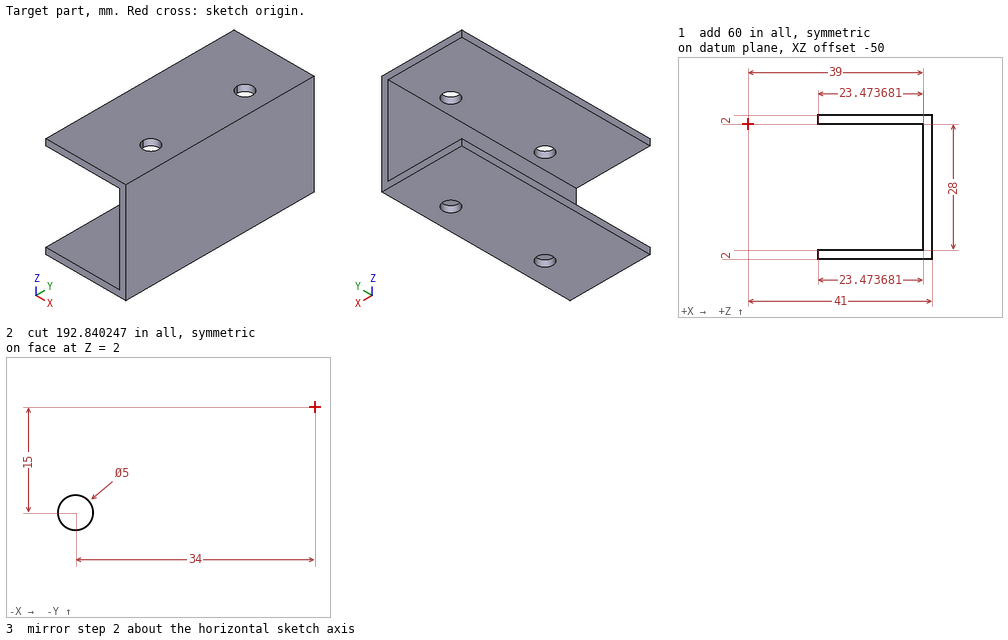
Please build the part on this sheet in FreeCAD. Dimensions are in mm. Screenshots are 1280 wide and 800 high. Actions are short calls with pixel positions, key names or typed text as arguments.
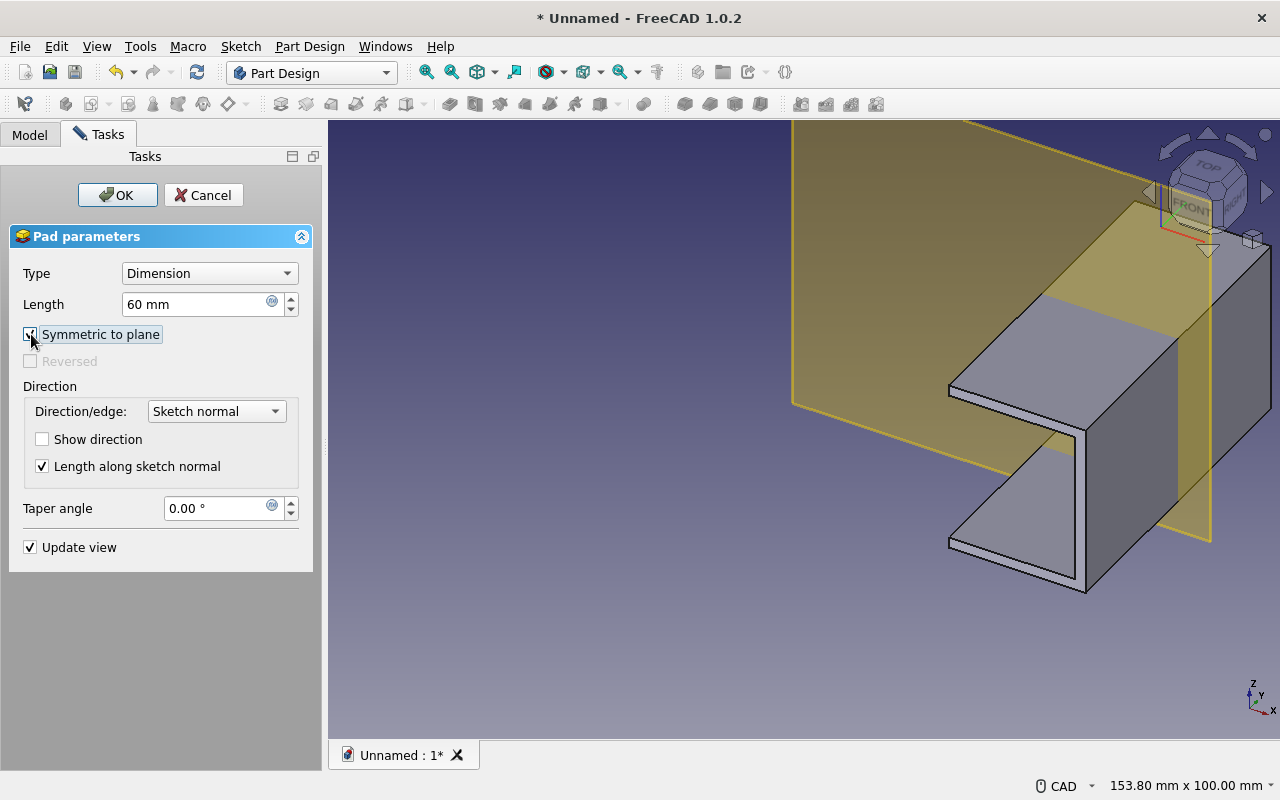
click(118, 195)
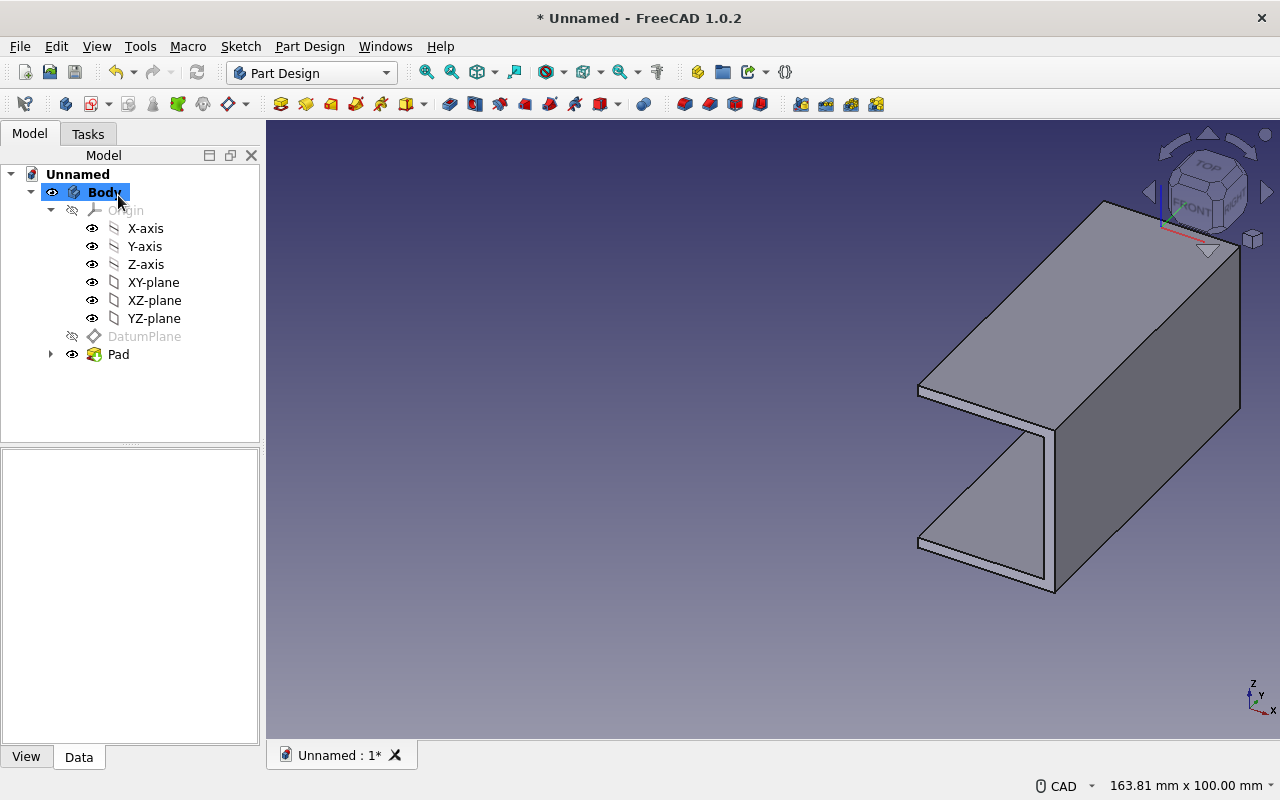
click(1106, 288)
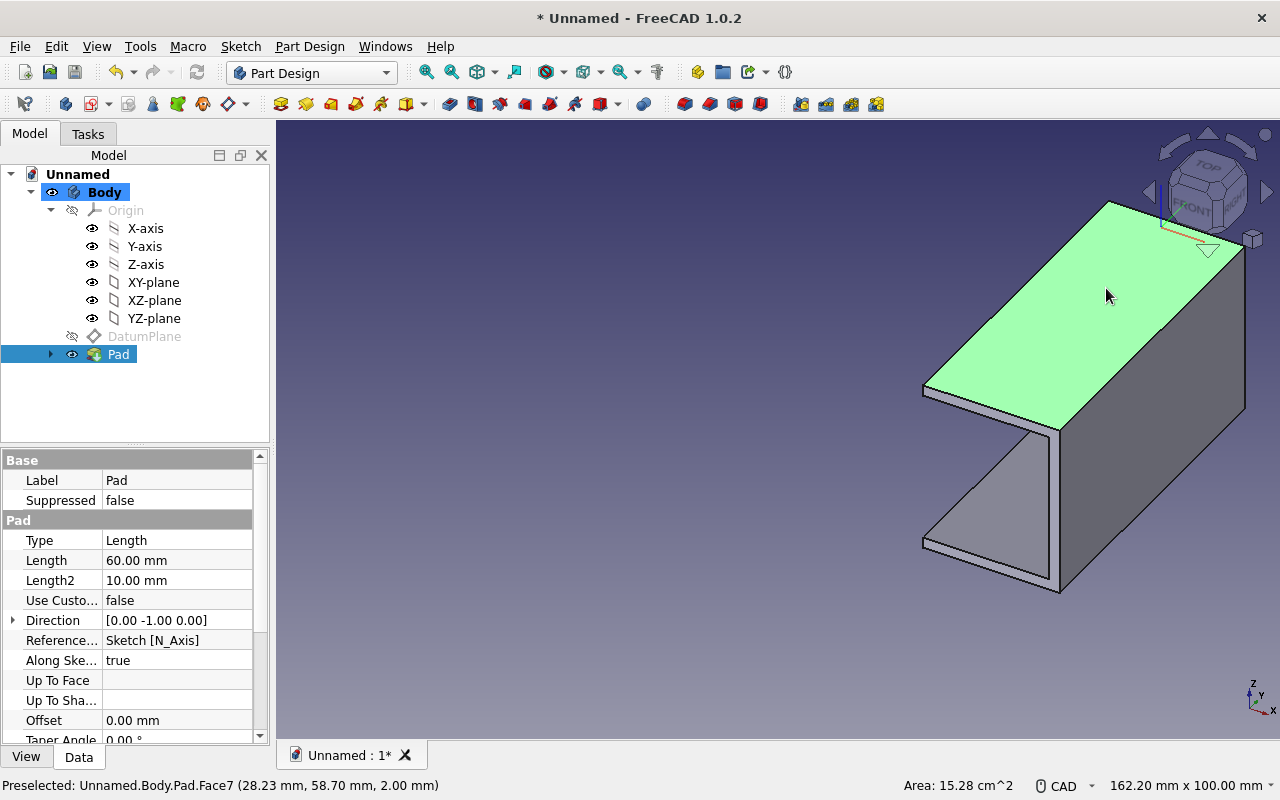
click(90, 104)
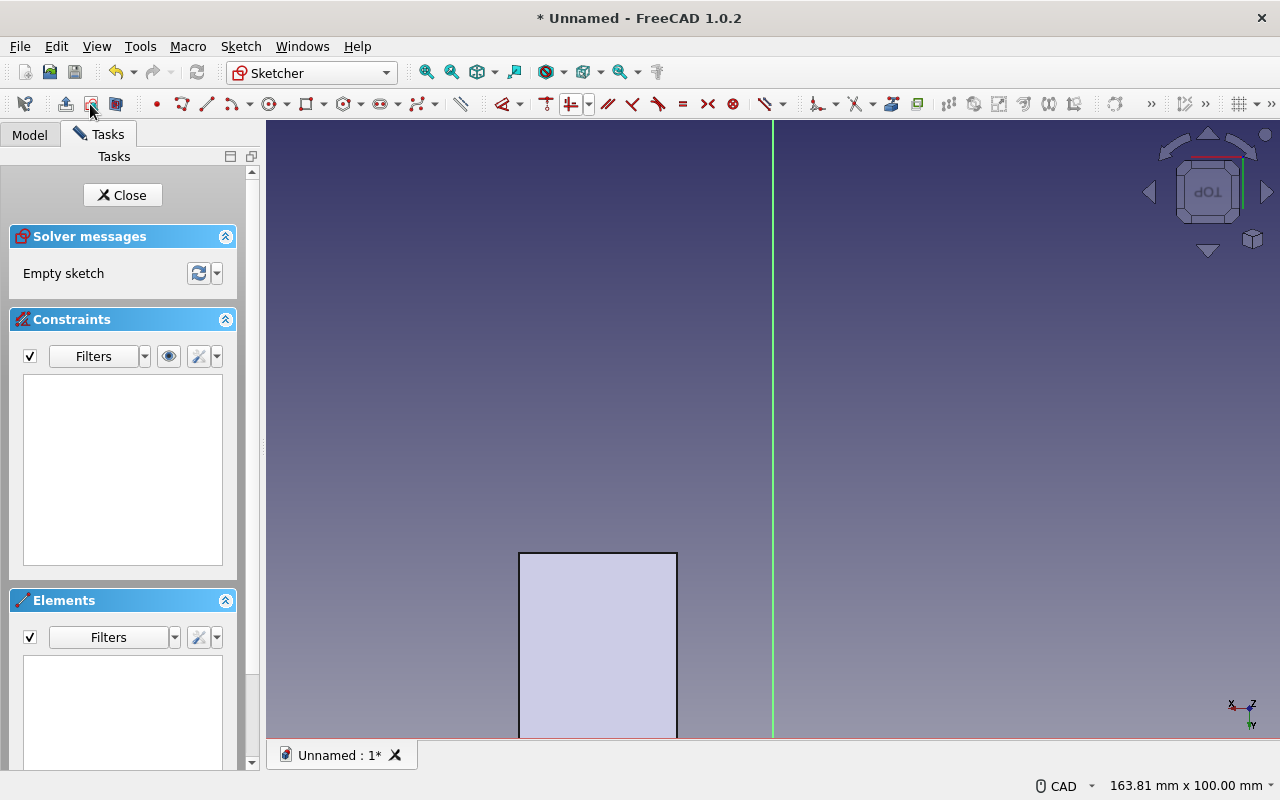
scroll(704, 430, down, 5)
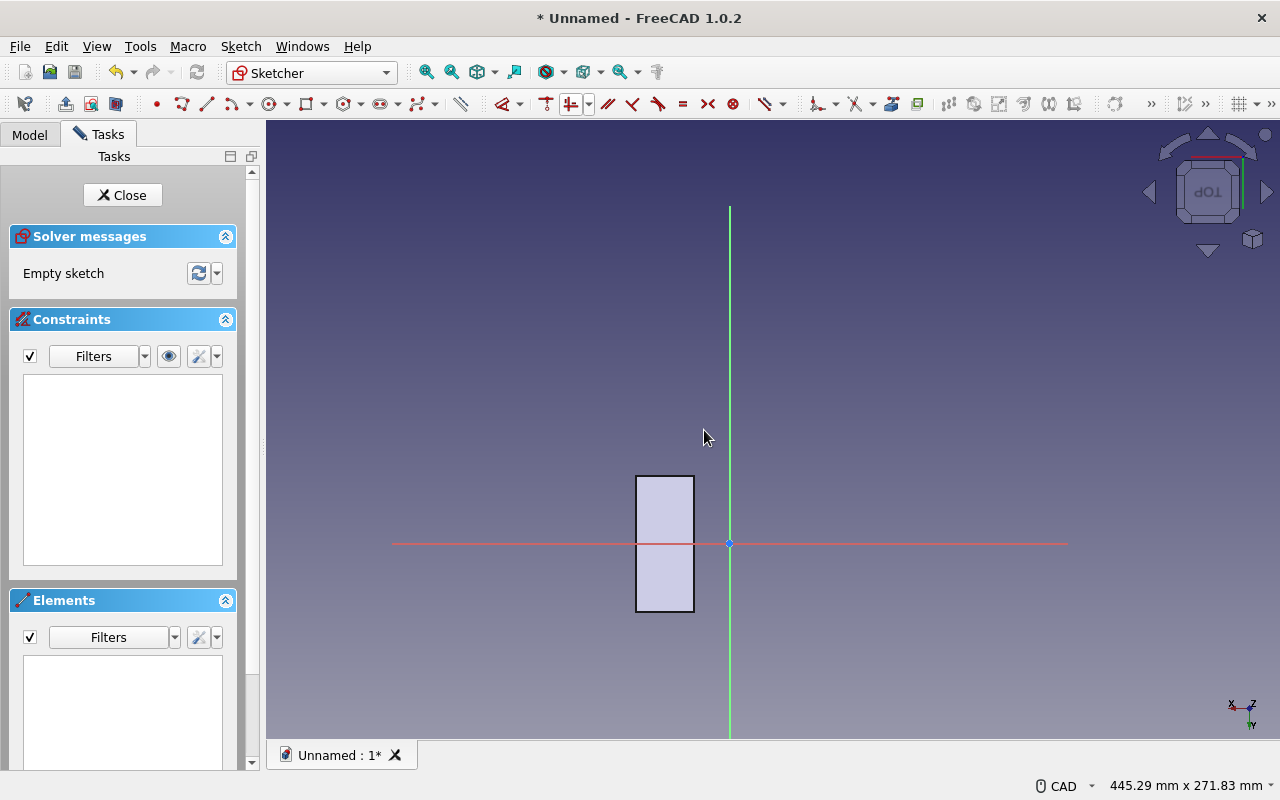
scroll(649, 586, up, 15)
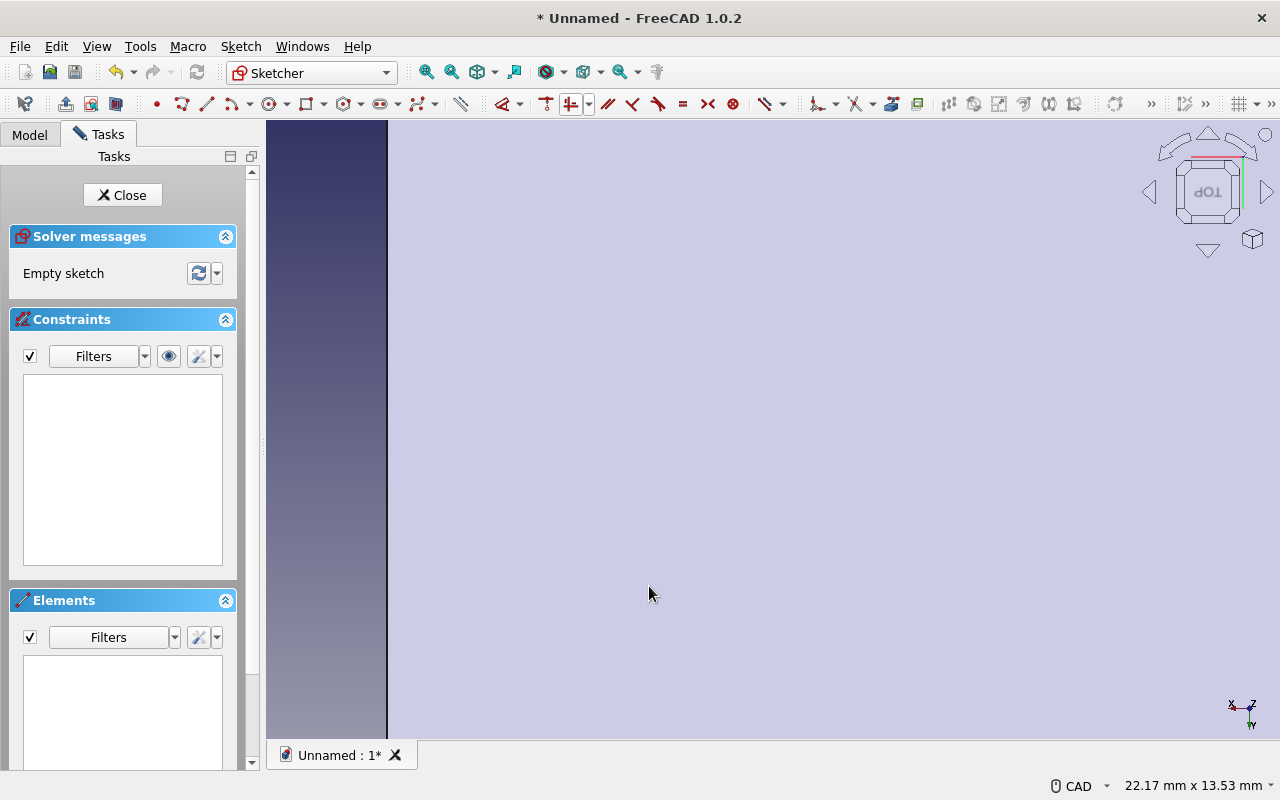
scroll(709, 395, up, 3)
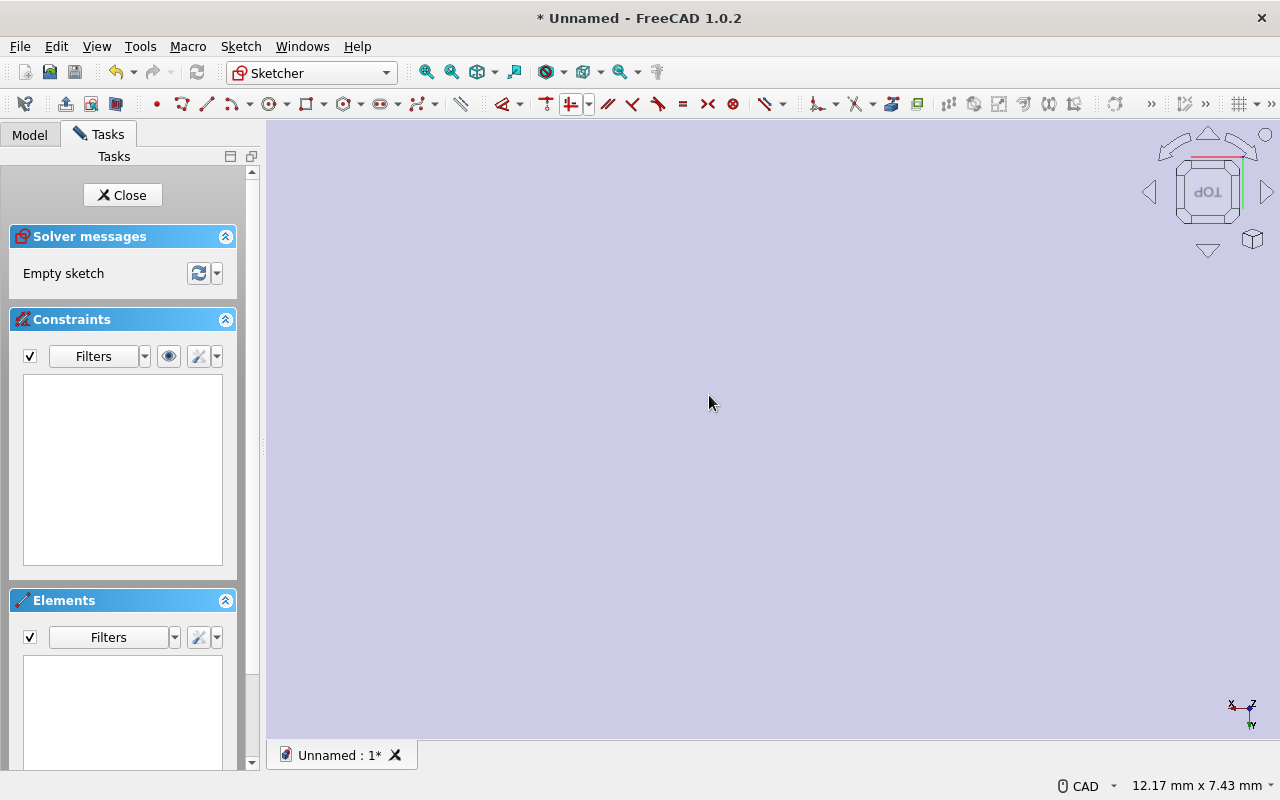
click(268, 104)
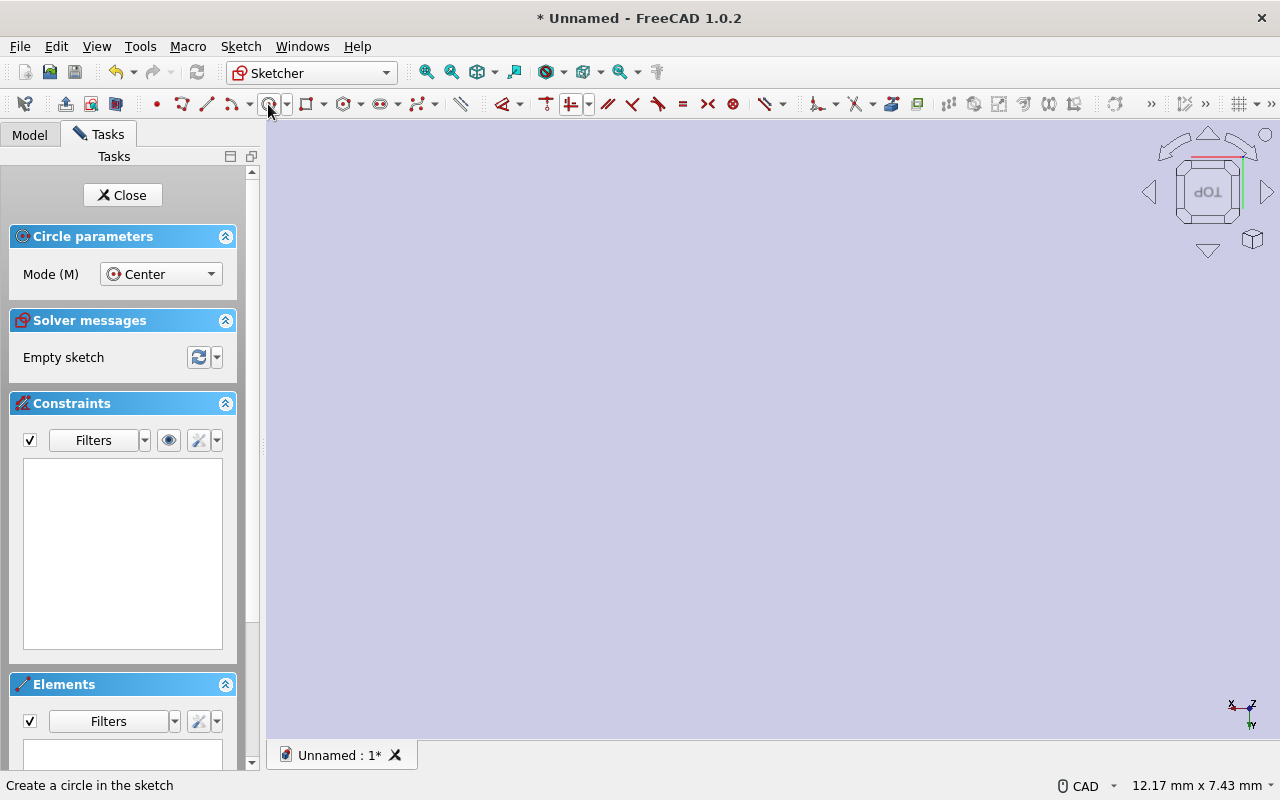
click(704, 429)
click(852, 282)
key(Escape)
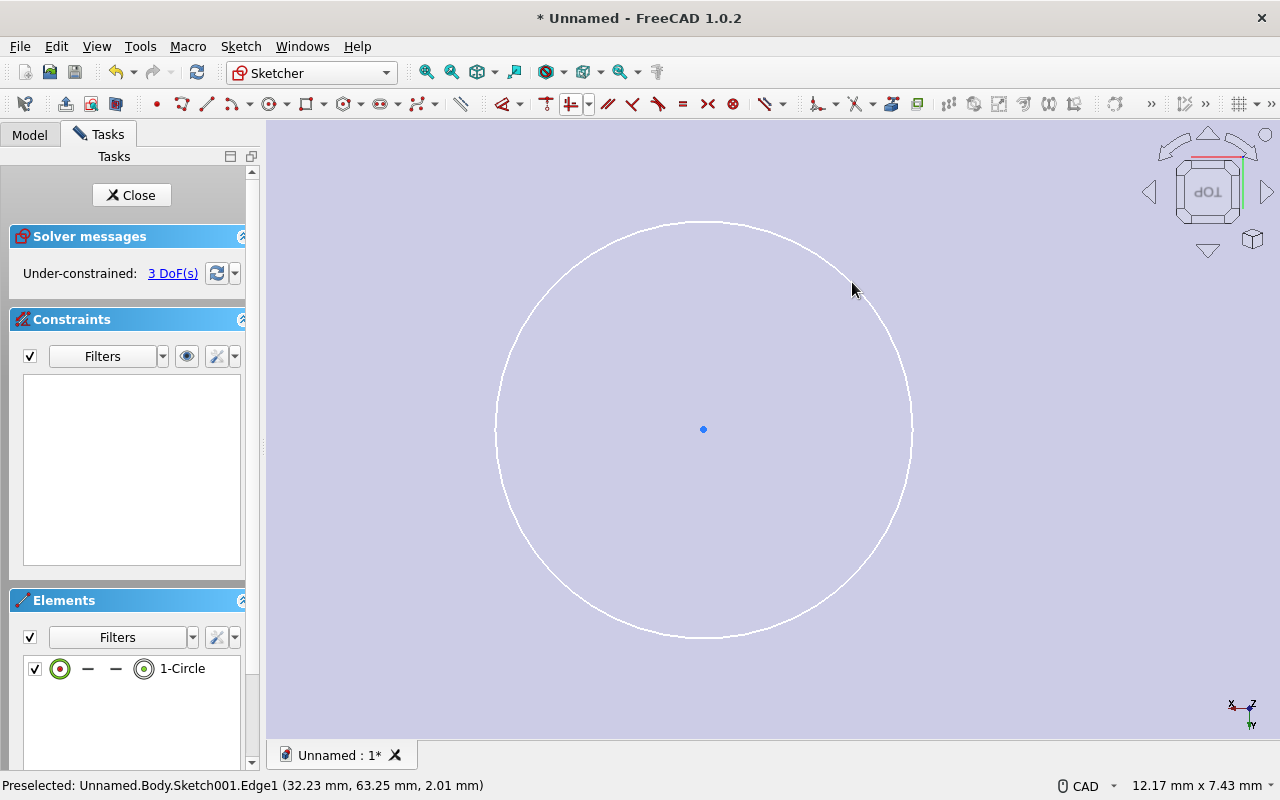
click(502, 104)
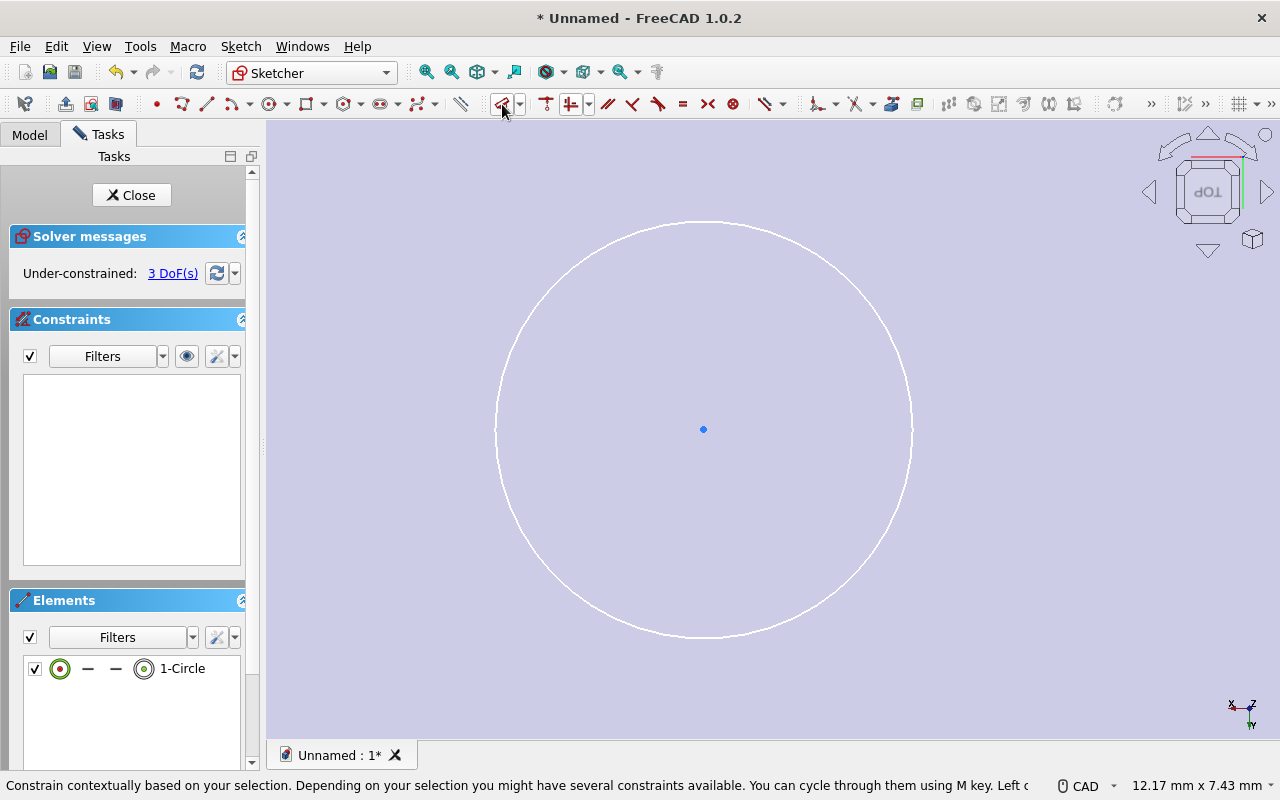
click(851, 282)
click(874, 259)